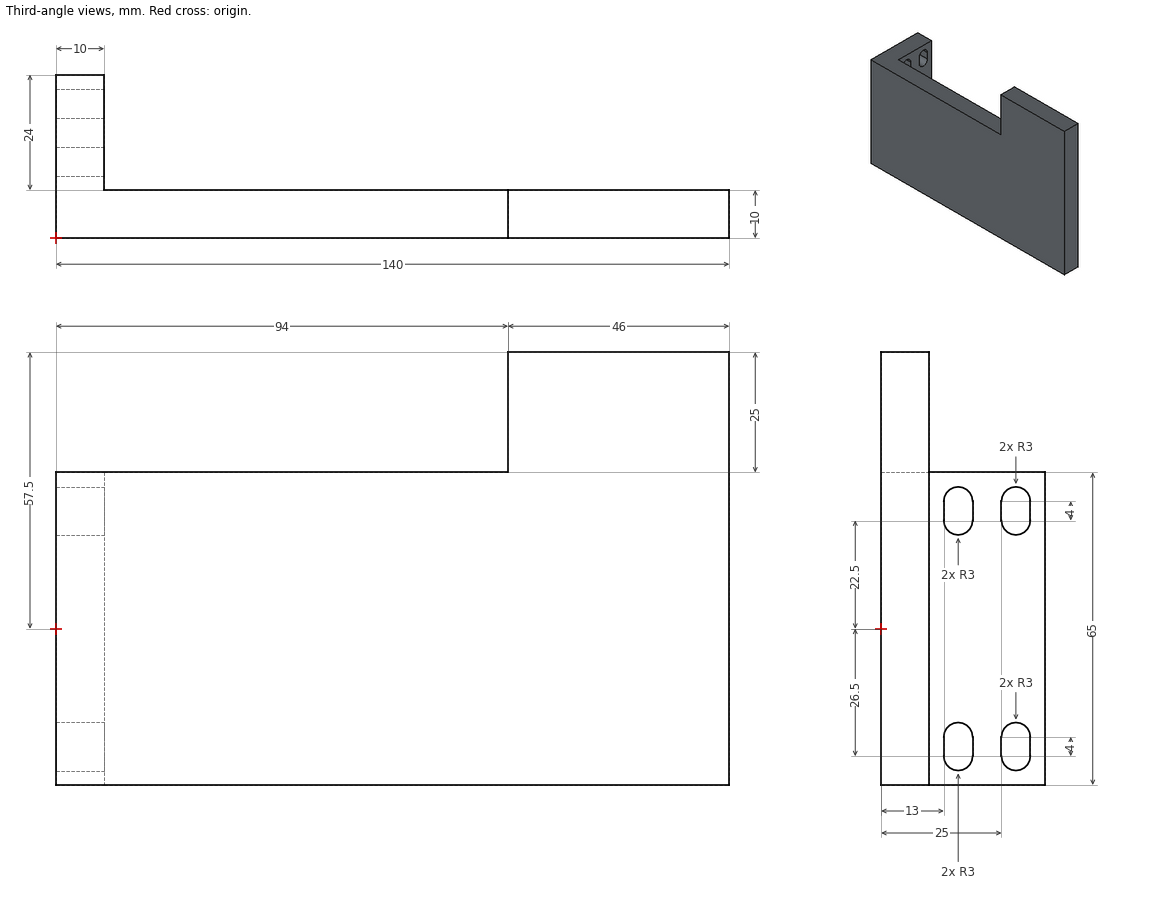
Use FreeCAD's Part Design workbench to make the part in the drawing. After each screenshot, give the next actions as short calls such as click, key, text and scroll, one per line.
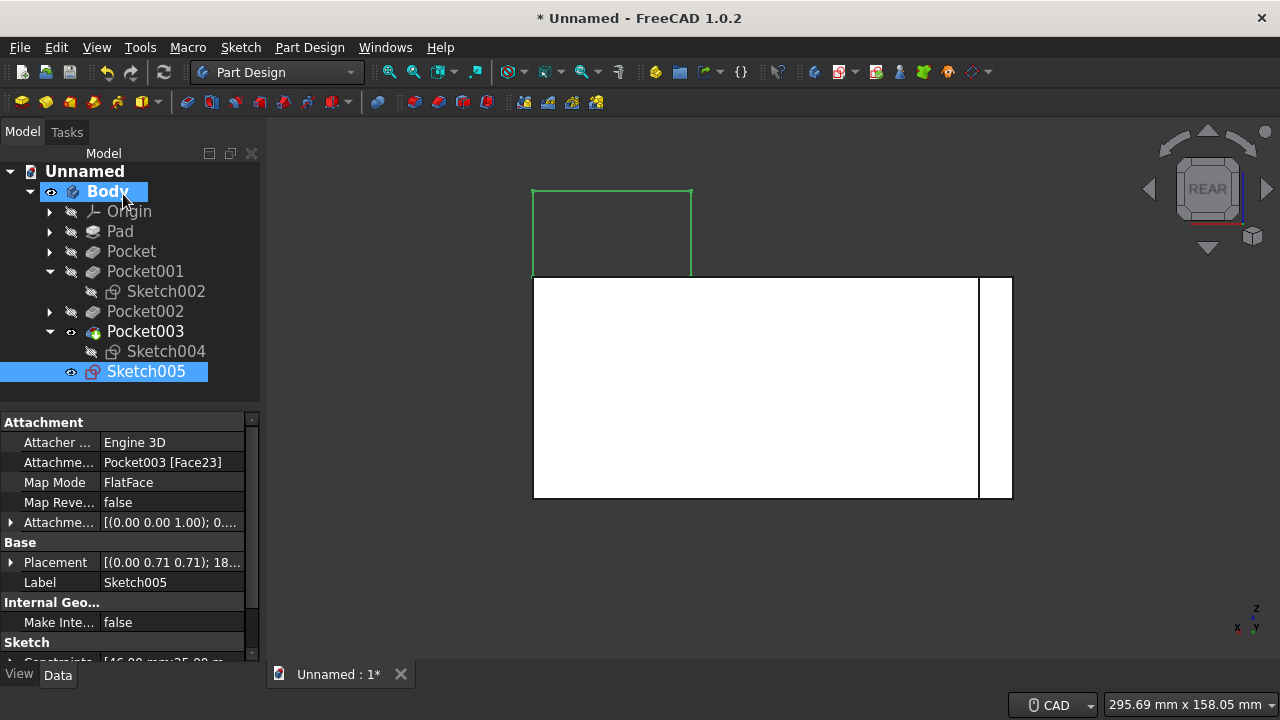
click(22, 102)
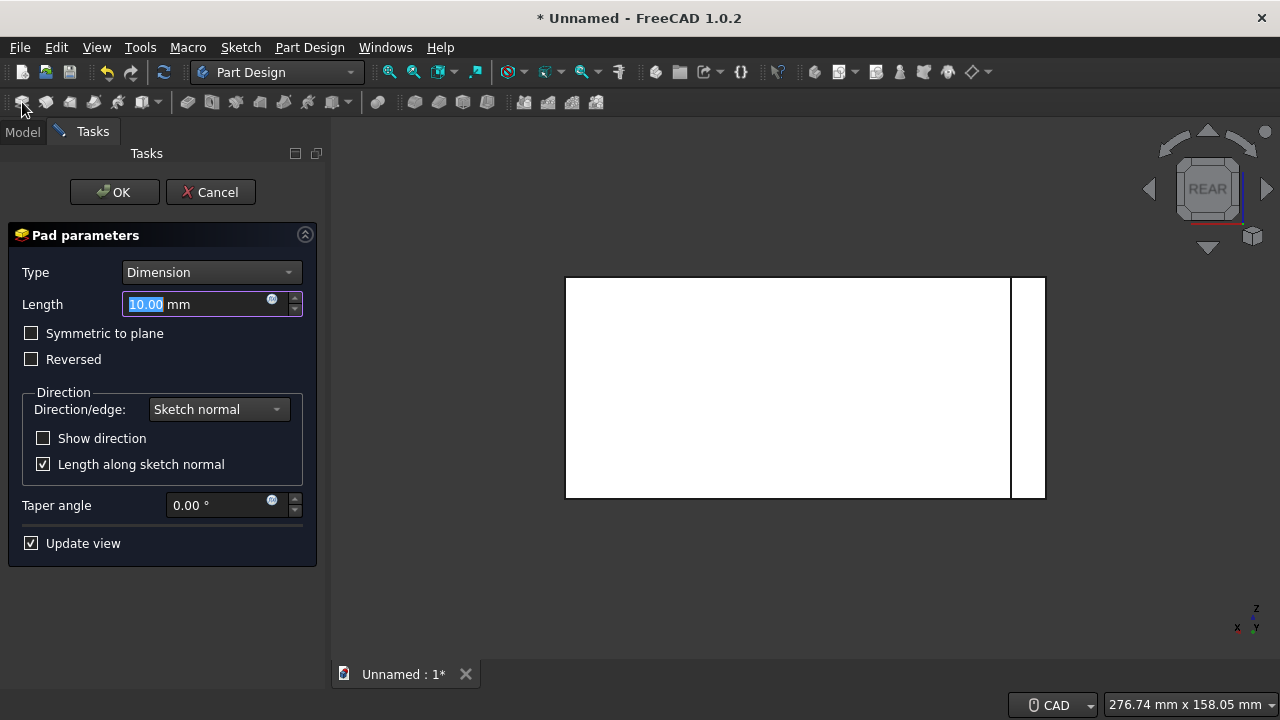
text(10)
key(Tab)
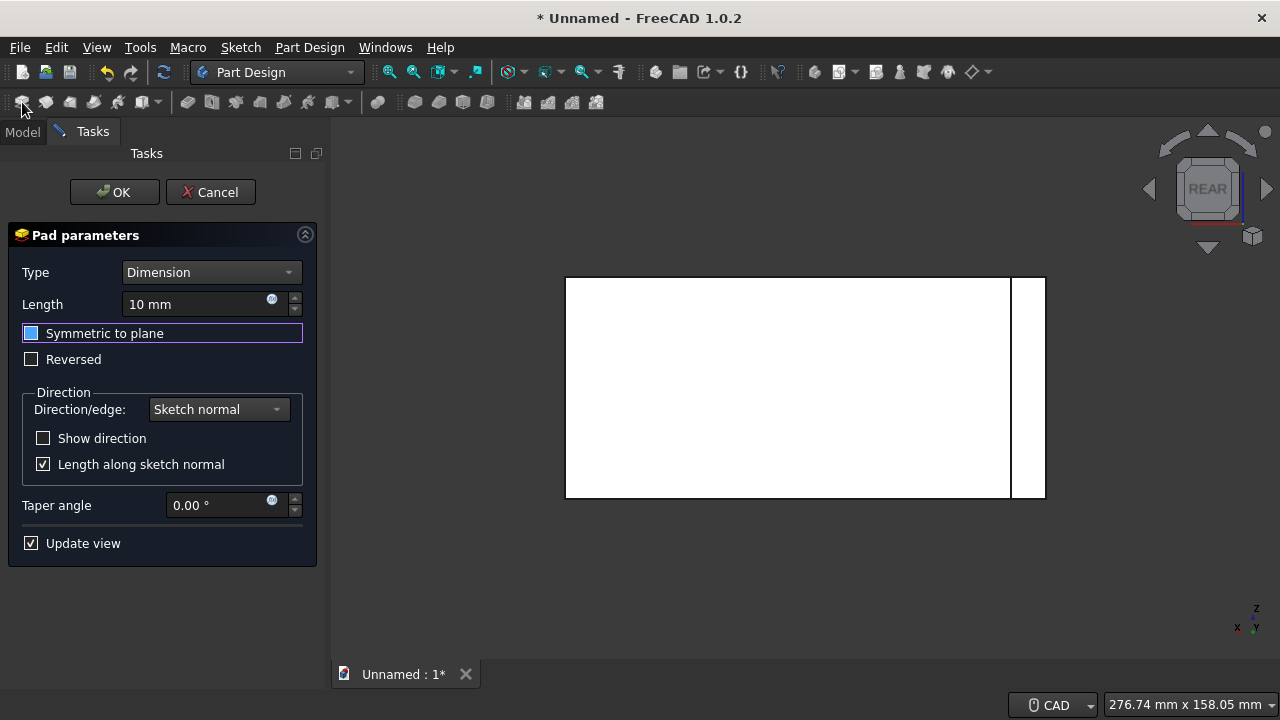
click(30, 359)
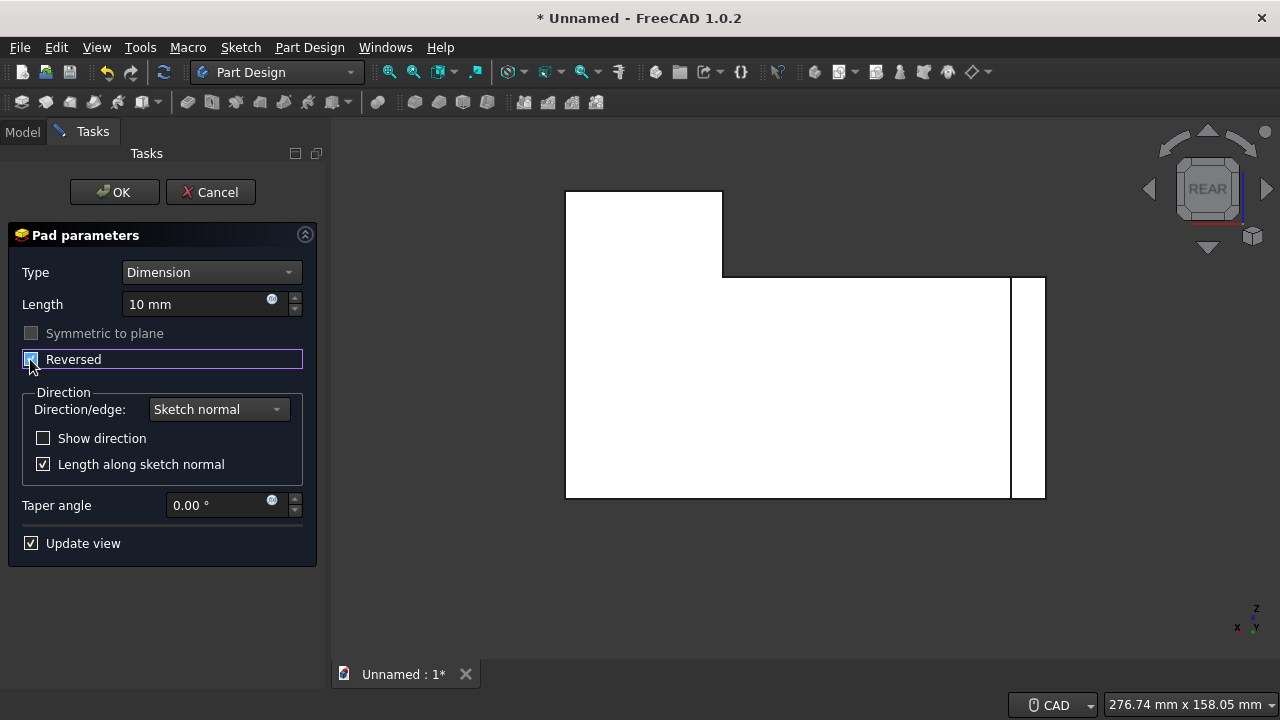
click(115, 192)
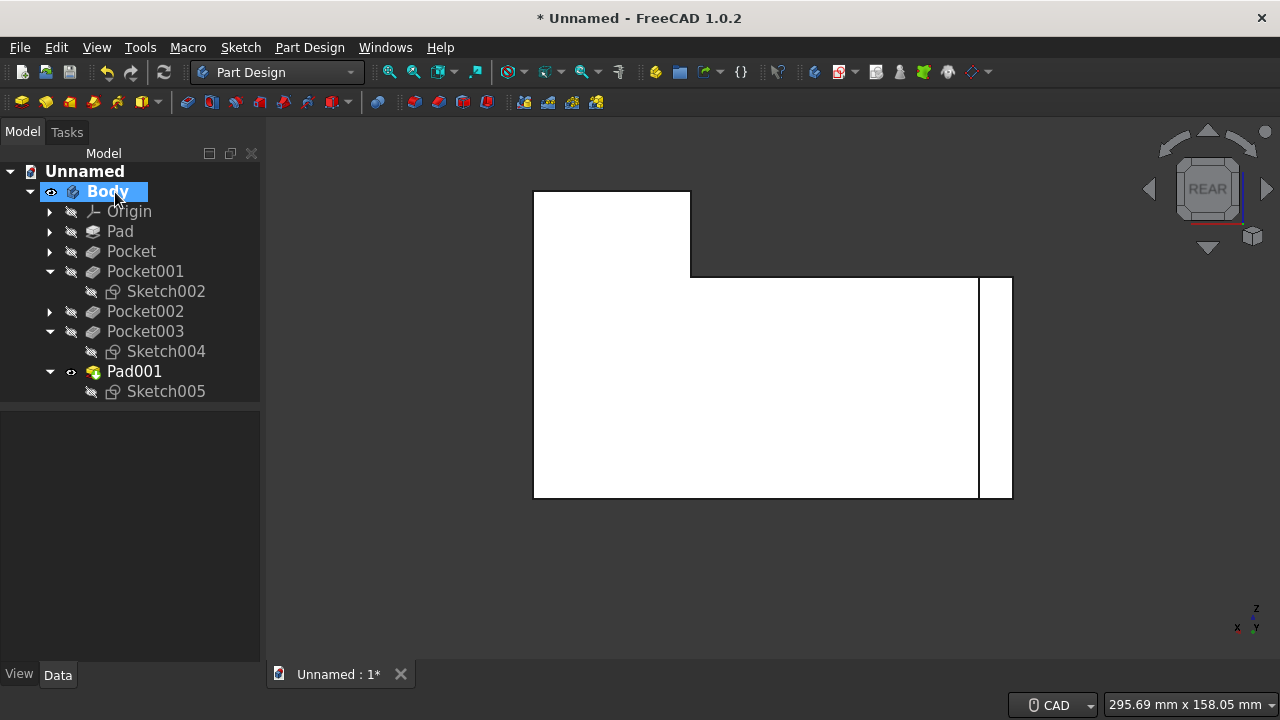
key(0)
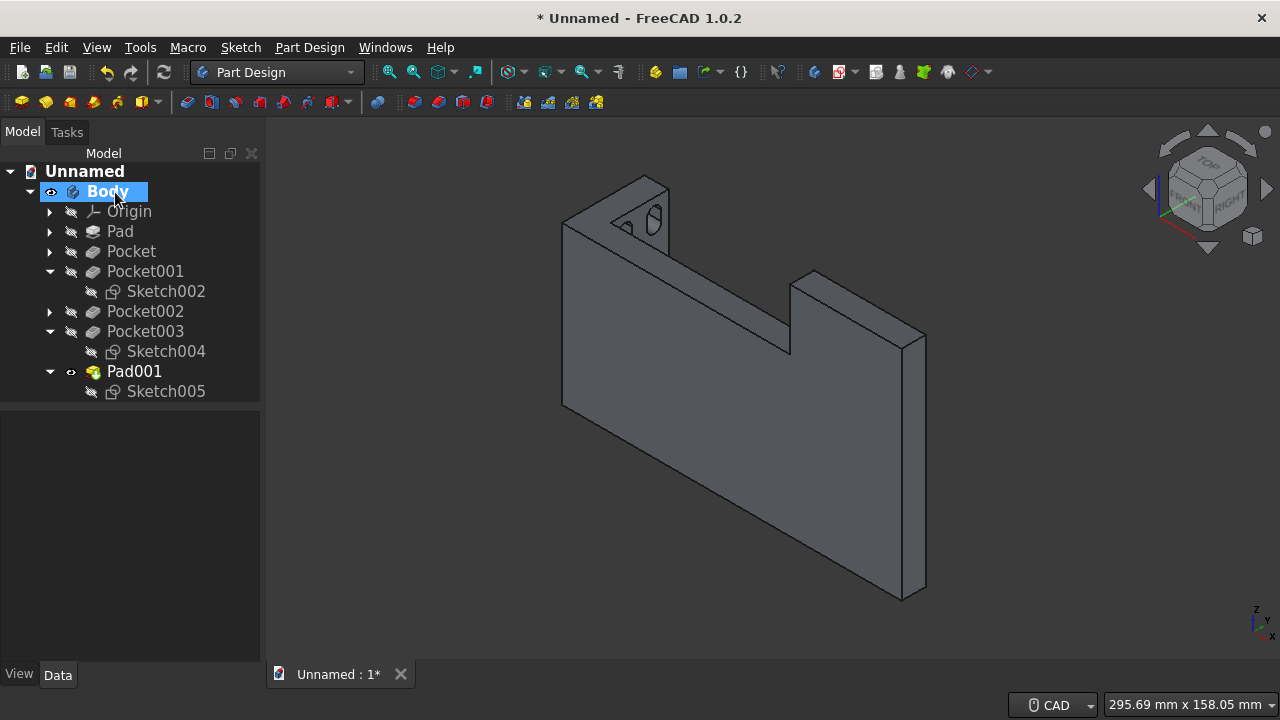
key(v)
key(f)